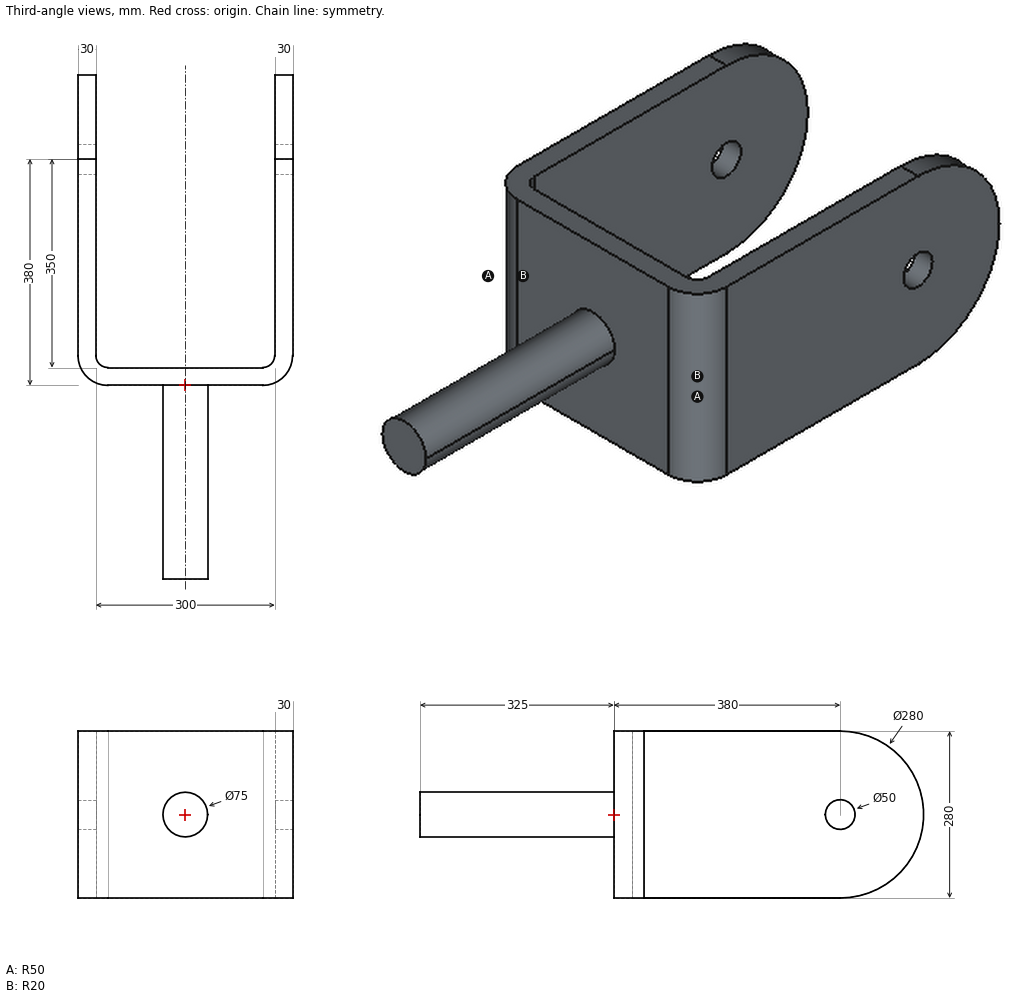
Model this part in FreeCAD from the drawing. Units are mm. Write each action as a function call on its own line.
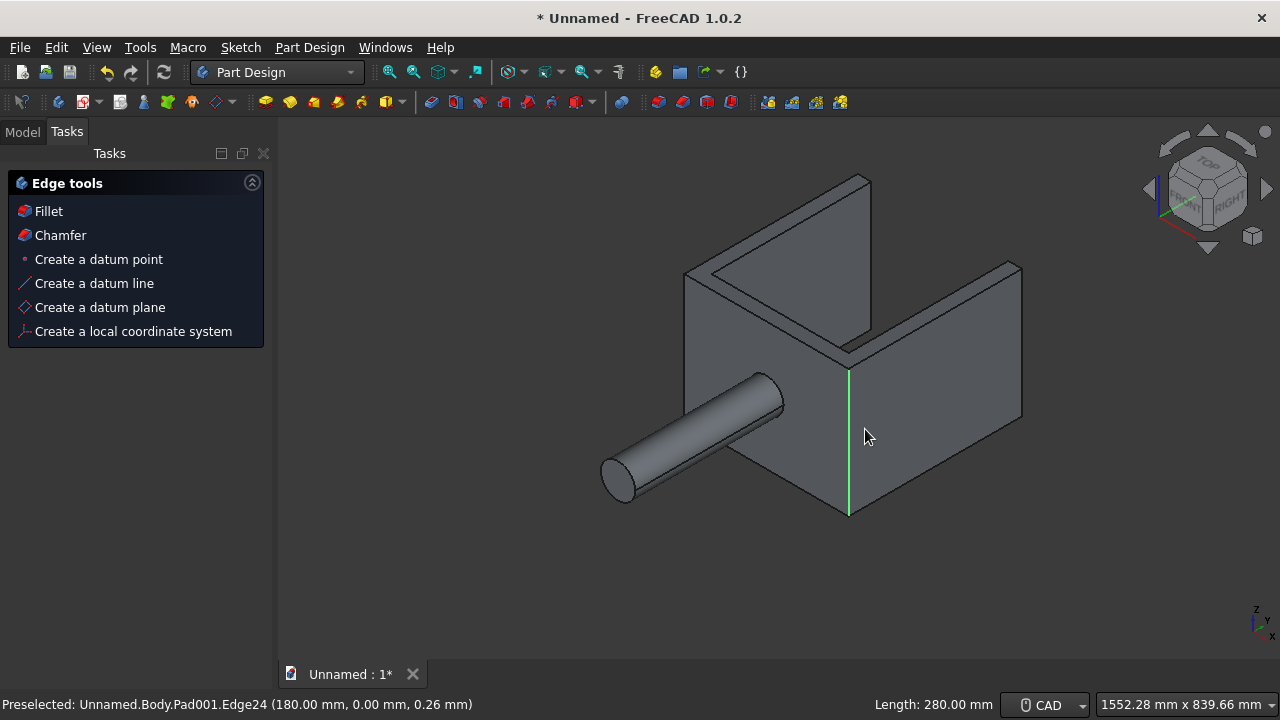
key(2)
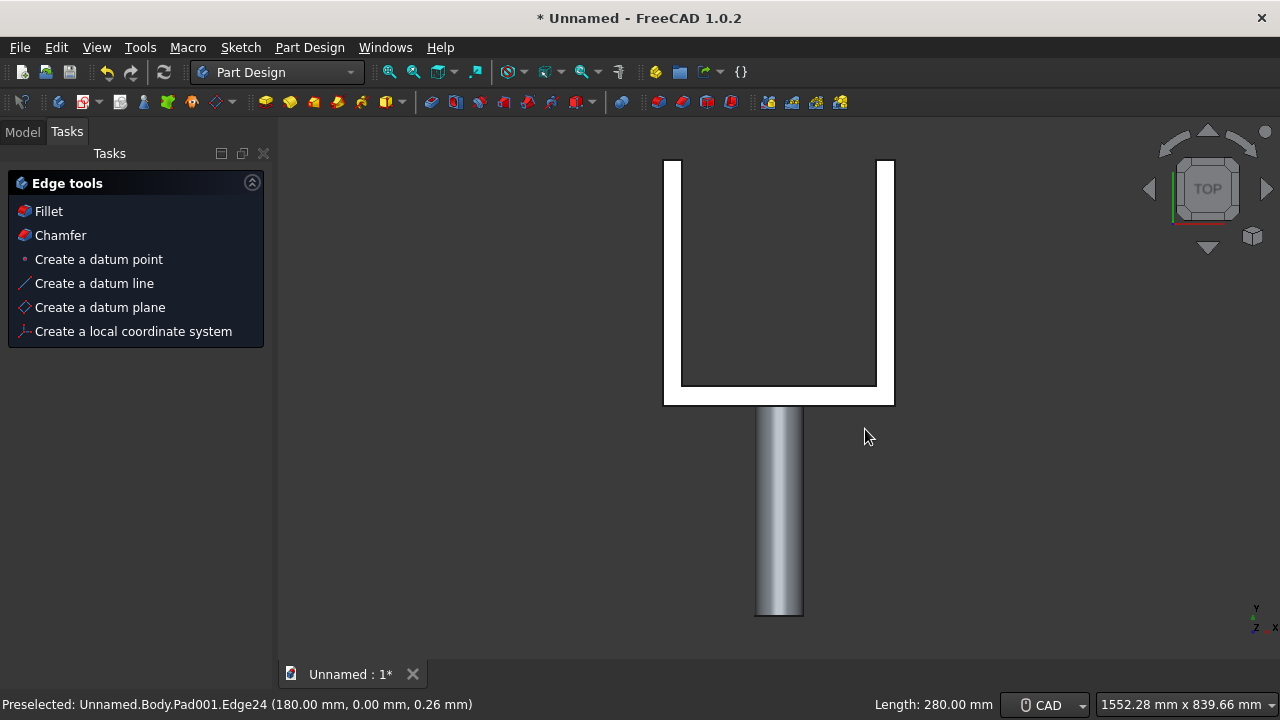
key(1)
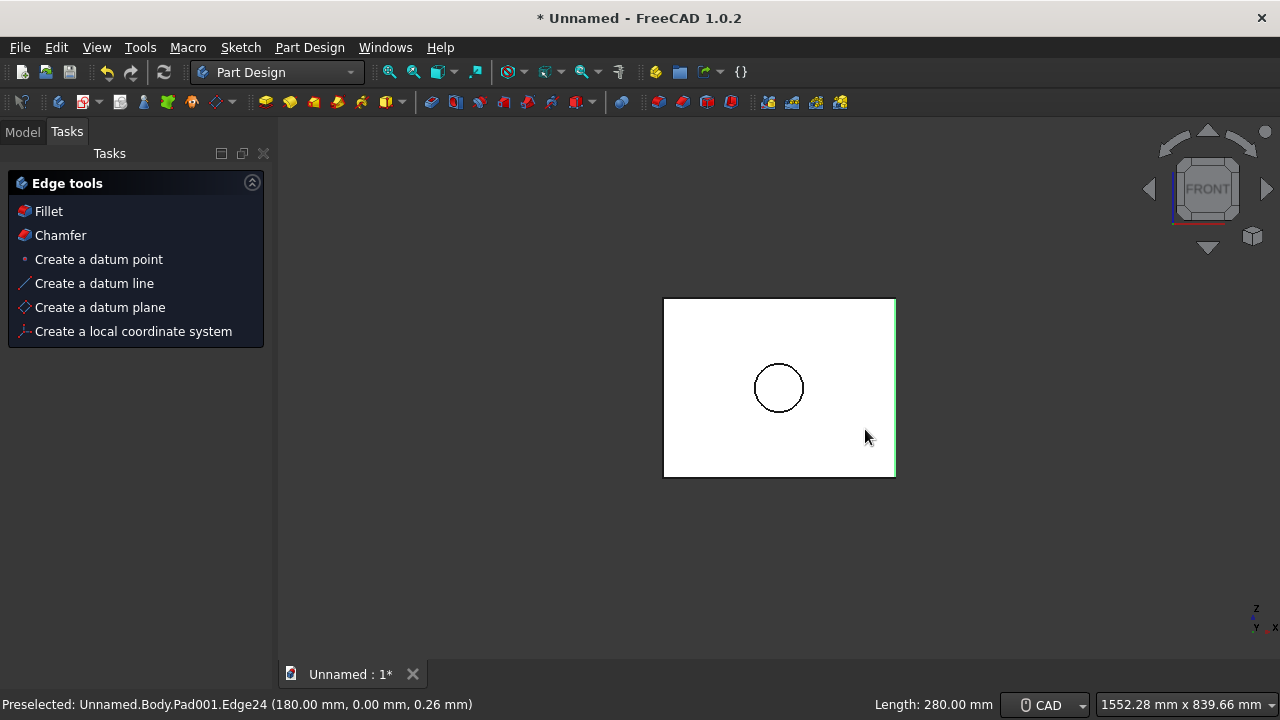
click(390, 72)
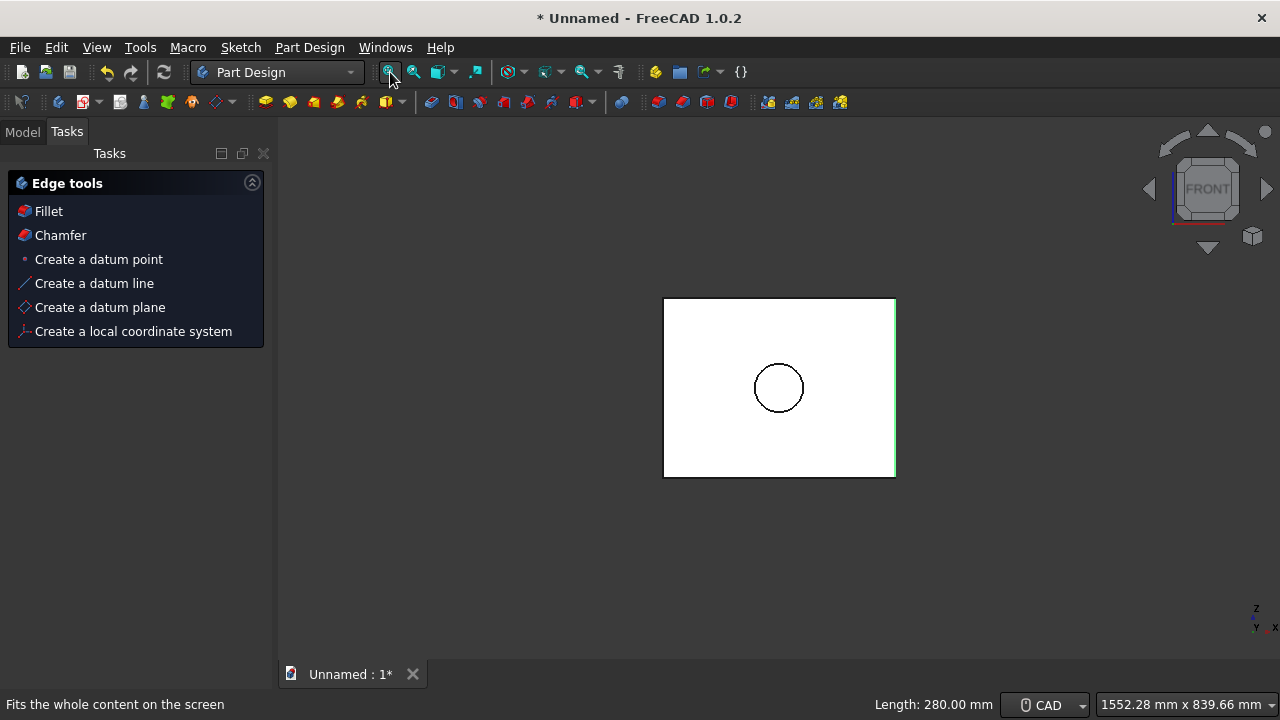
click(663, 387, ctrl)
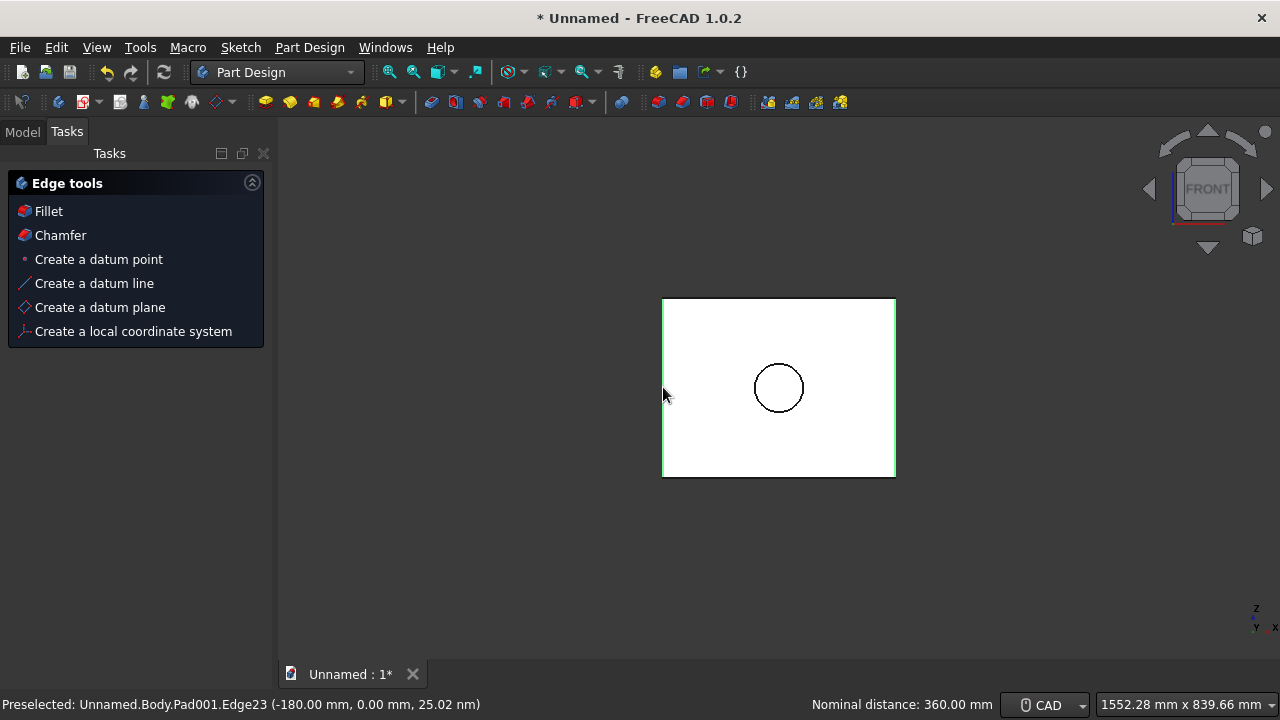
click(660, 102)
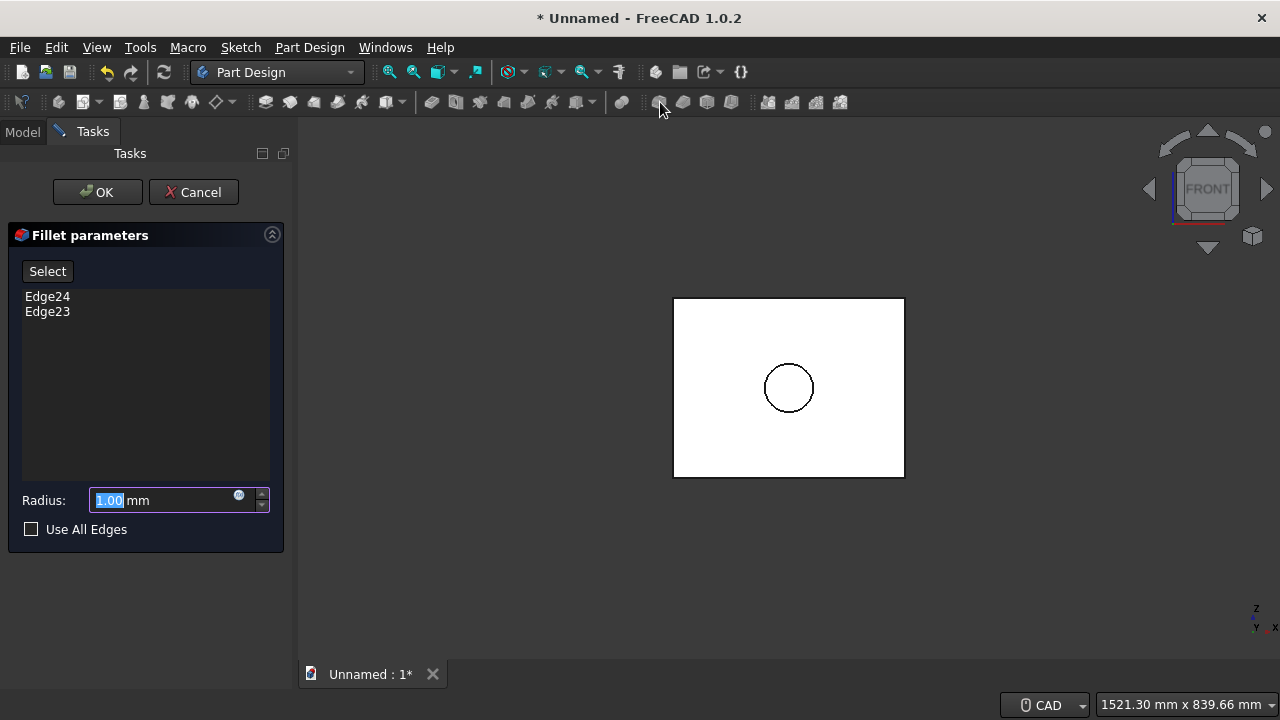
text(50)
key(Tab)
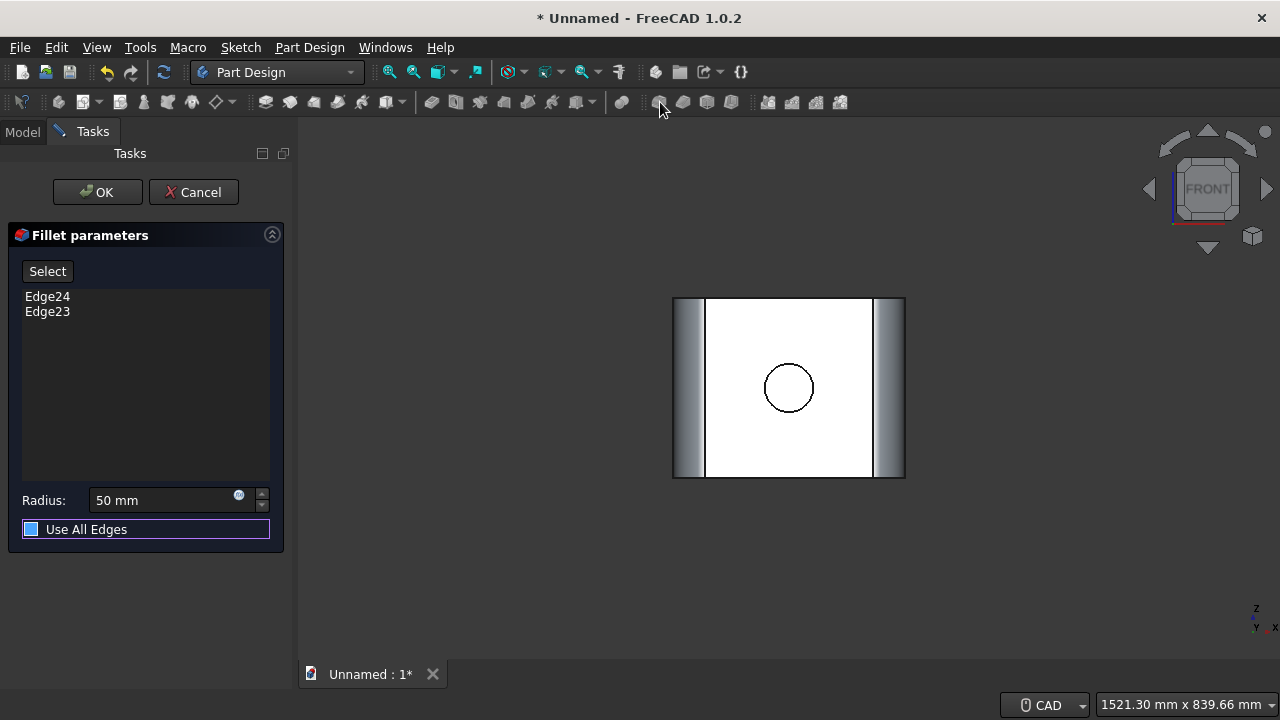
click(98, 192)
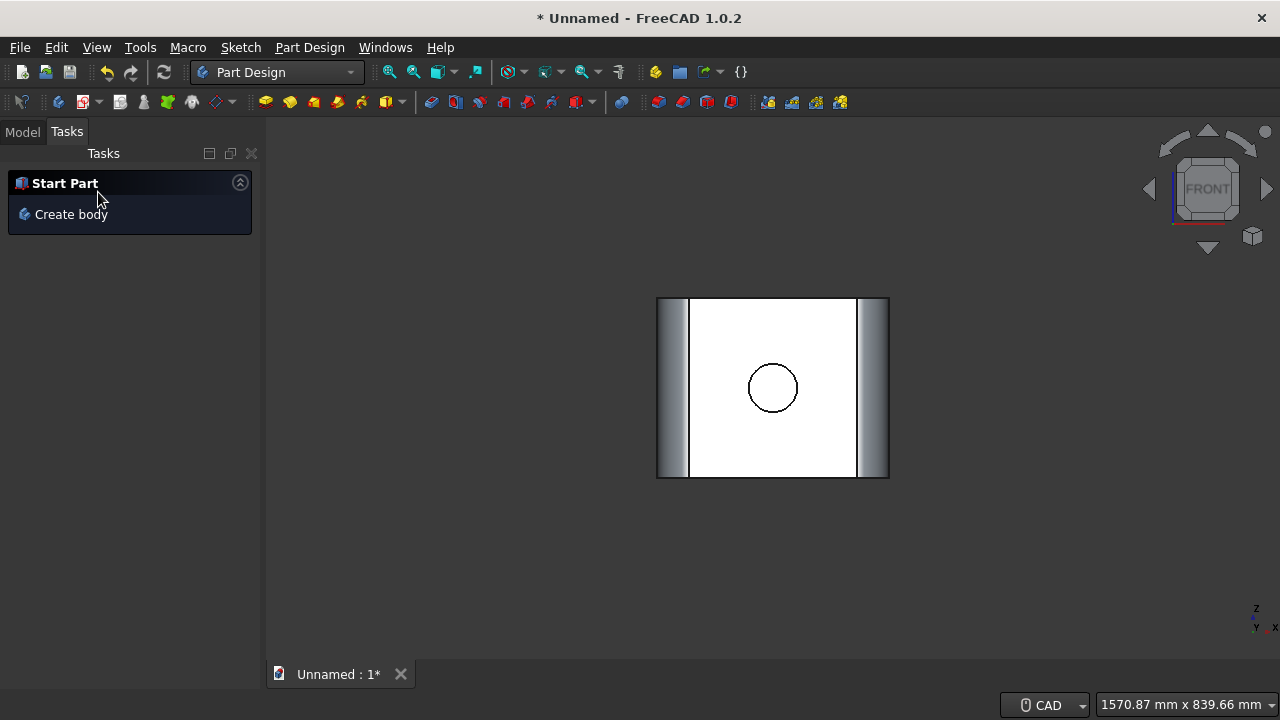
click(390, 72)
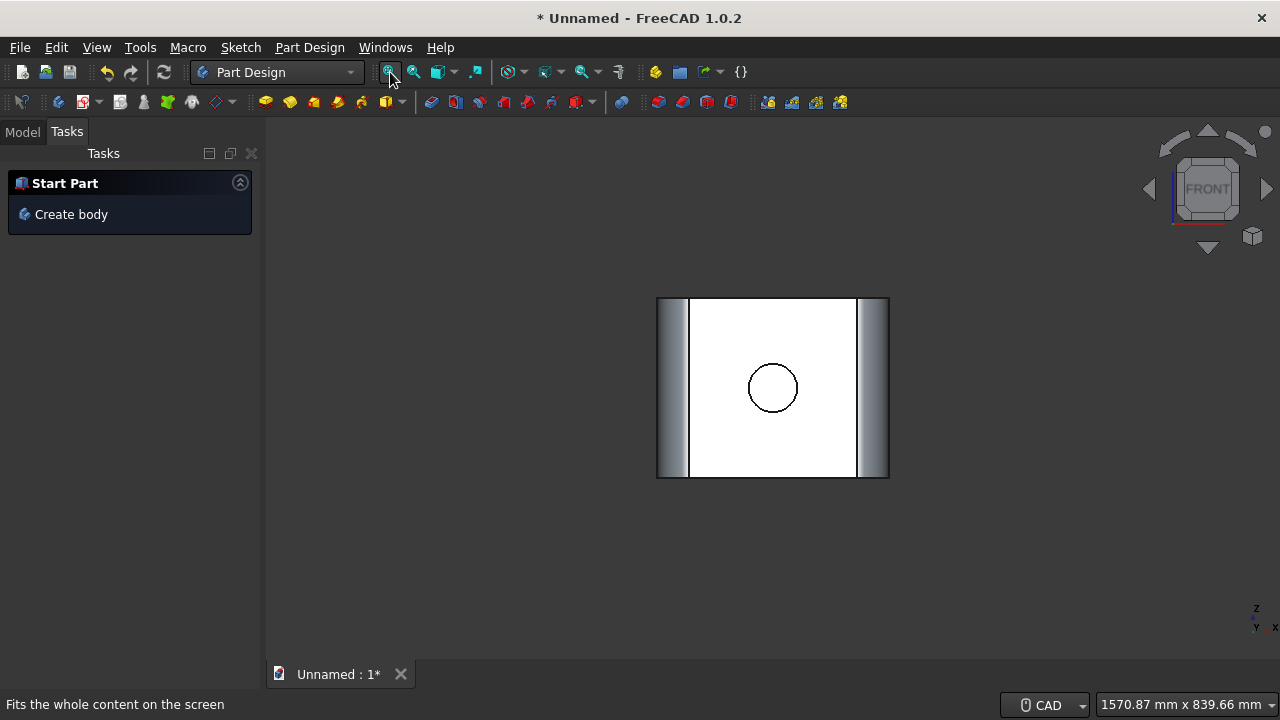
key(0)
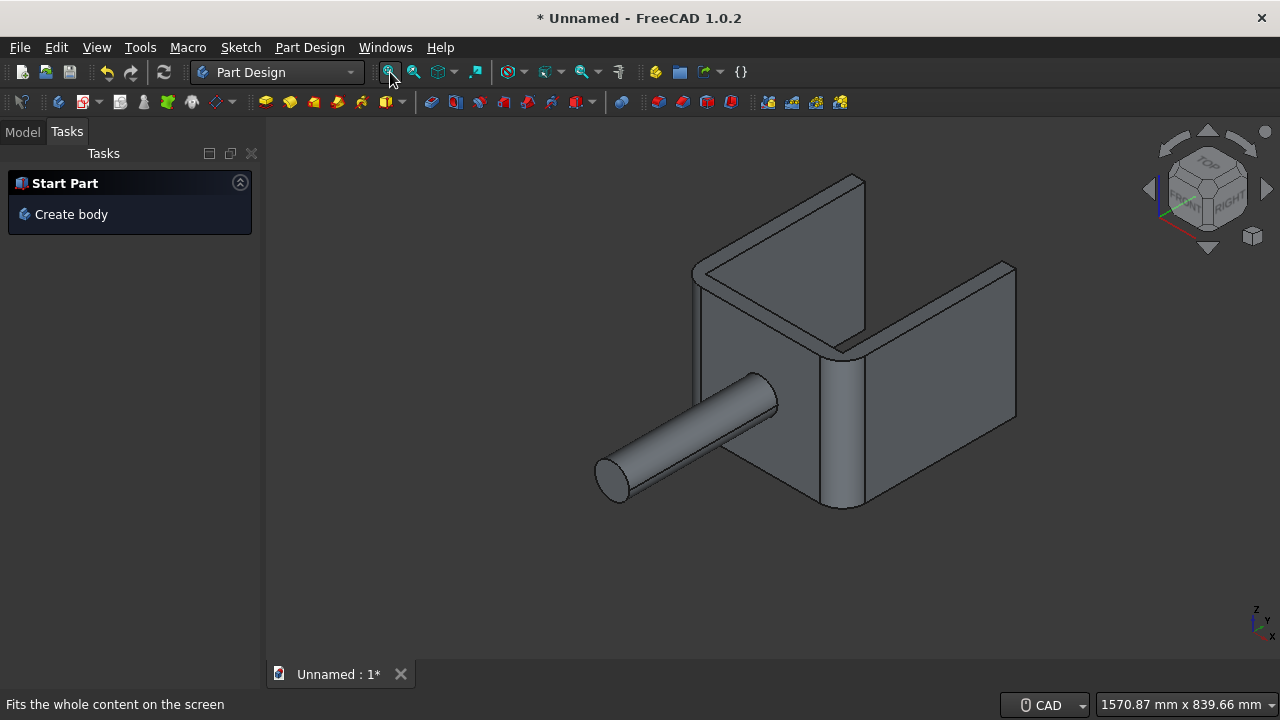
key(2)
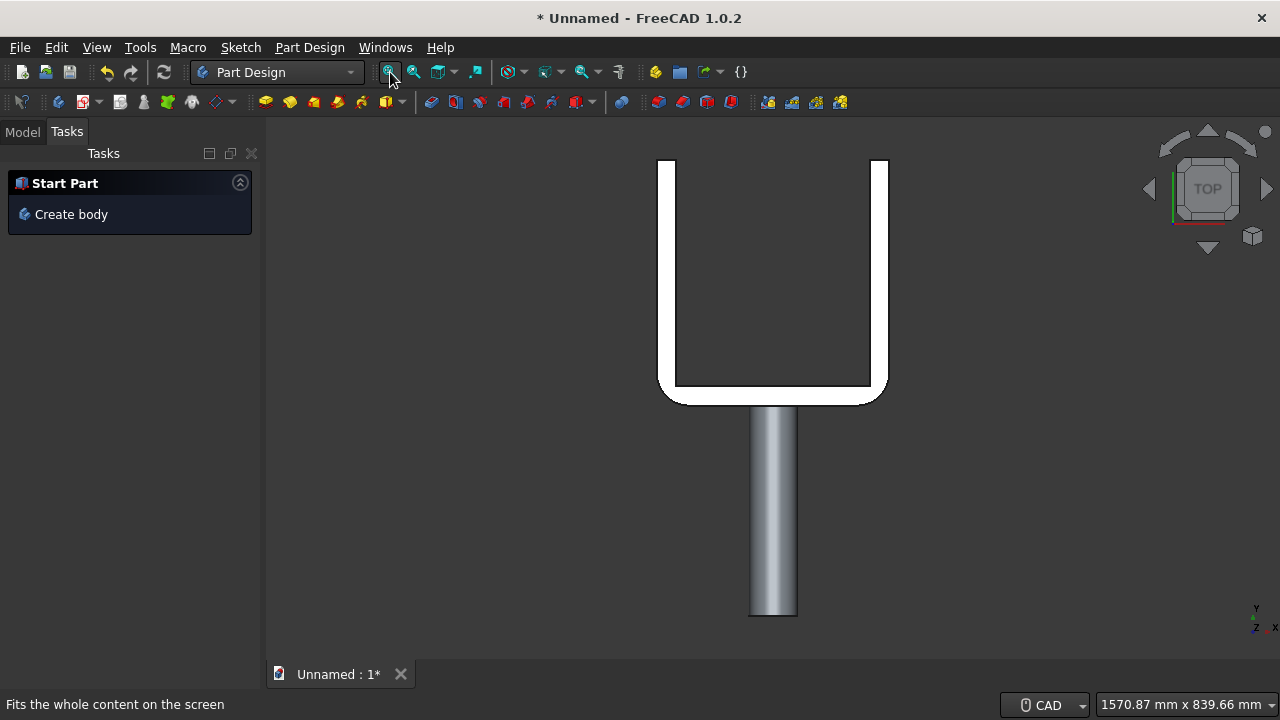
key(1)